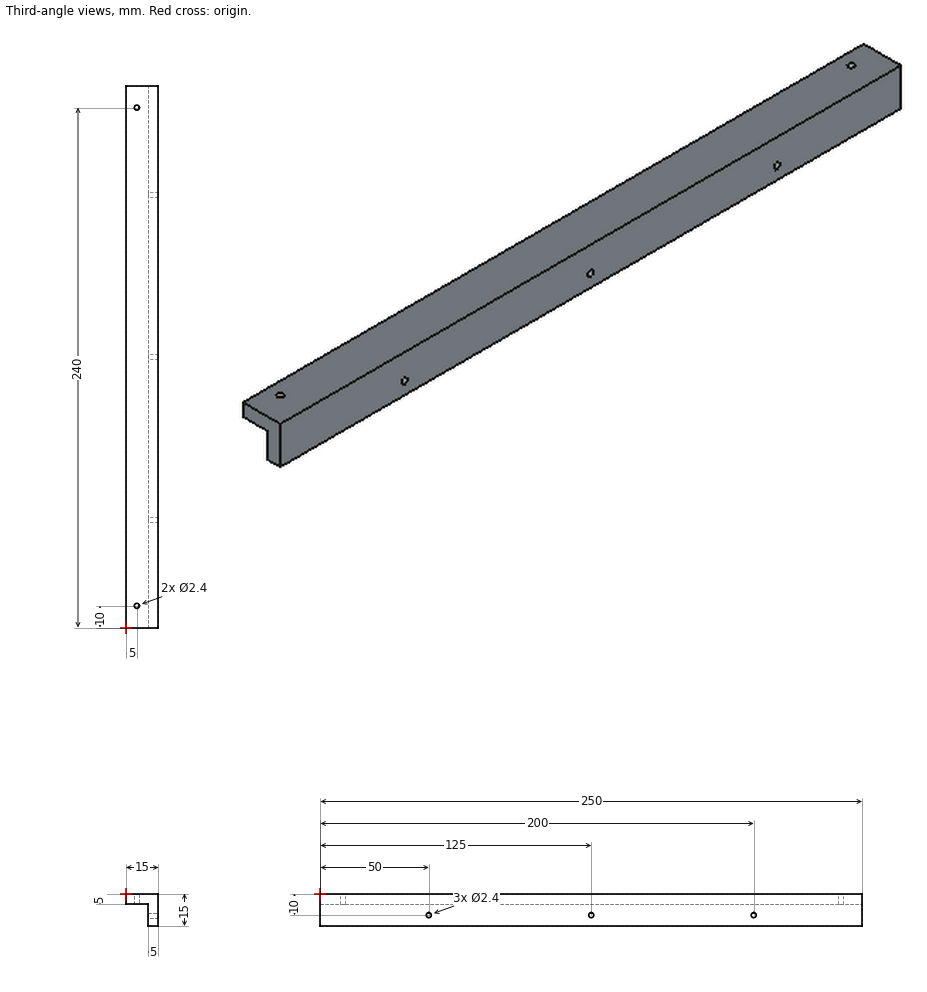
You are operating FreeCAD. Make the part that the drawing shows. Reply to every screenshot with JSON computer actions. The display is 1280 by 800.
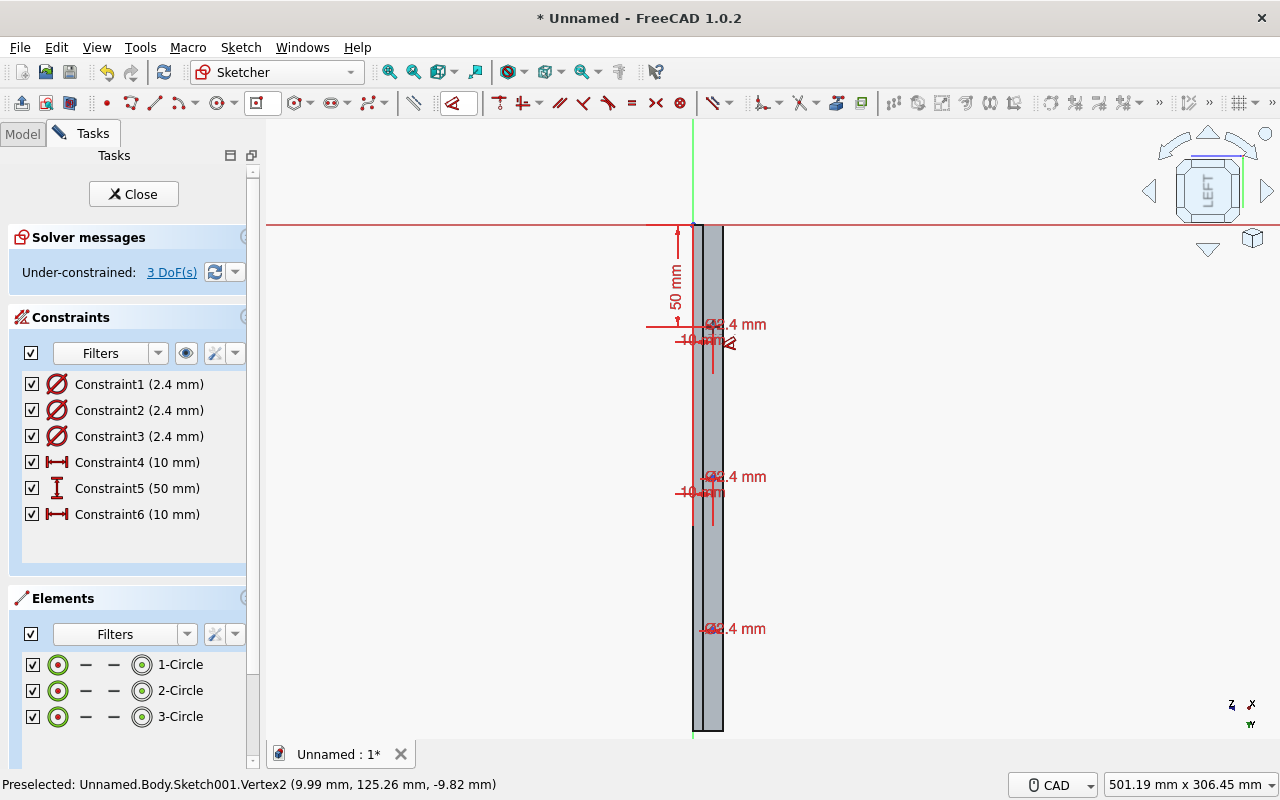
{"action": "scroll", "coordinate": [713, 631], "scroll_direction": "up", "scroll_amount": 4}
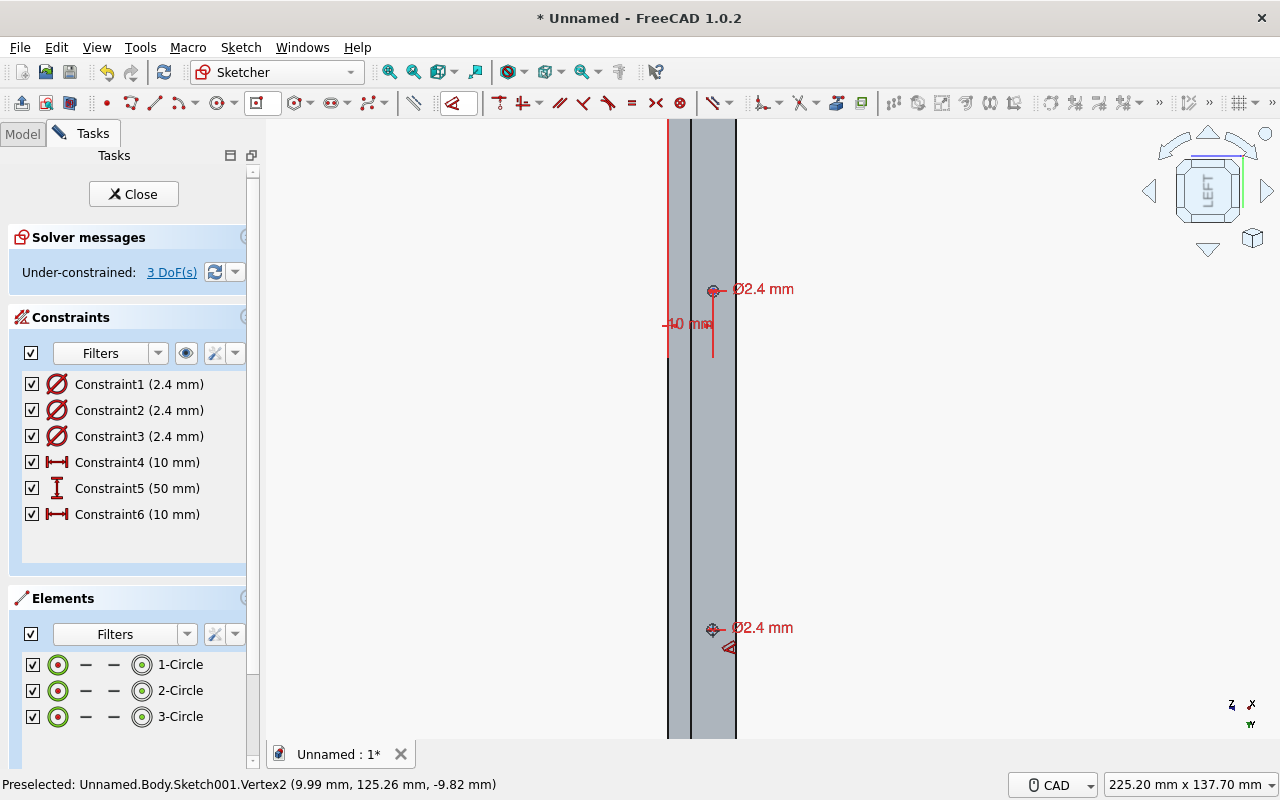
{"action": "left_click", "coordinate": [712, 630]}
{"action": "left_click", "coordinate": [690, 664]}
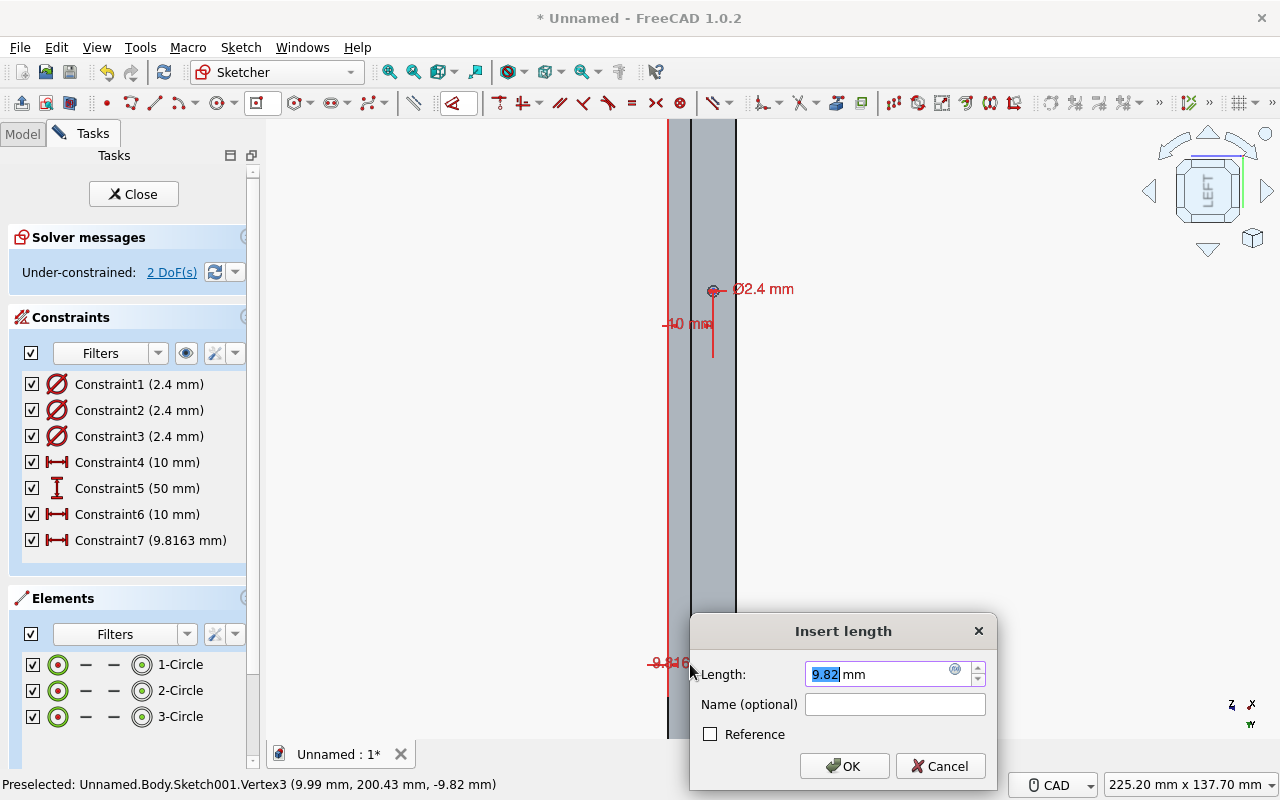
{"action": "type", "text": "10"}
{"action": "key", "text": "Return"}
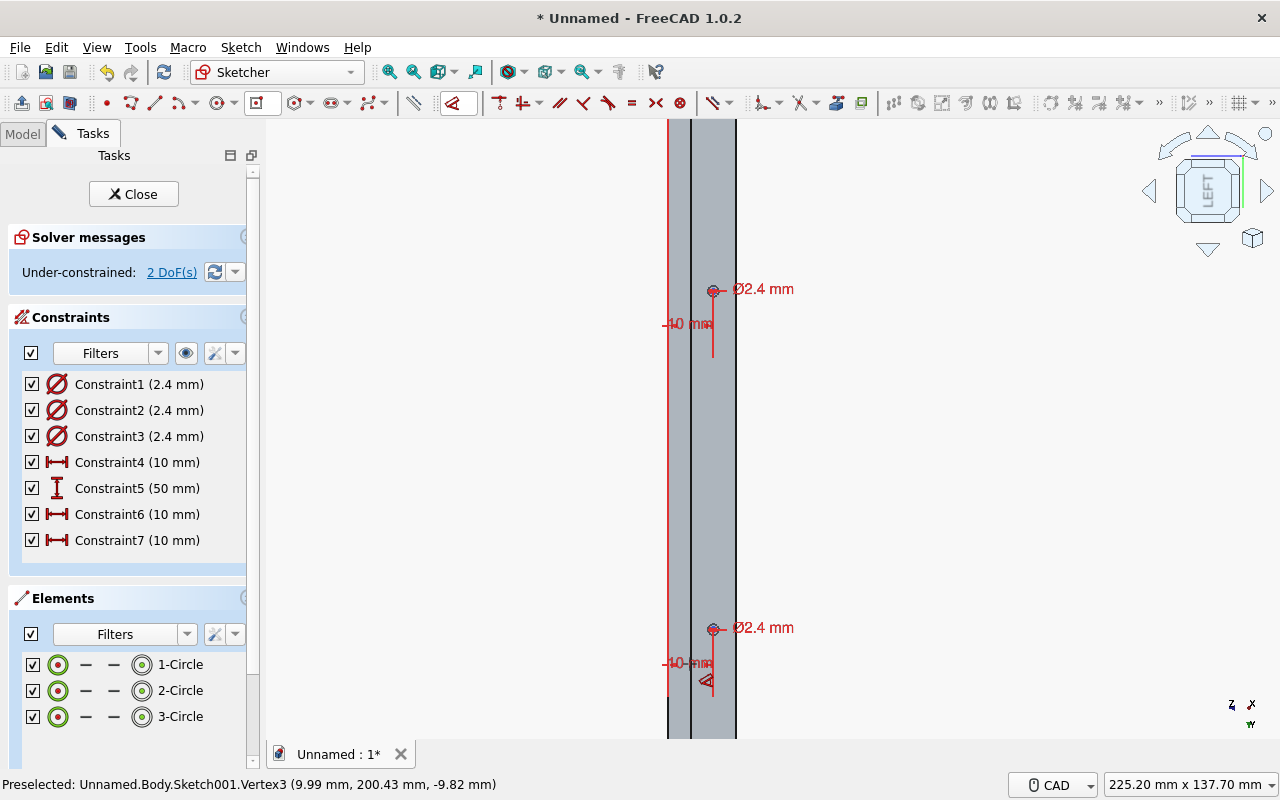
{"action": "left_click", "coordinate": [713, 291]}
{"action": "left_click", "coordinate": [634, 219]}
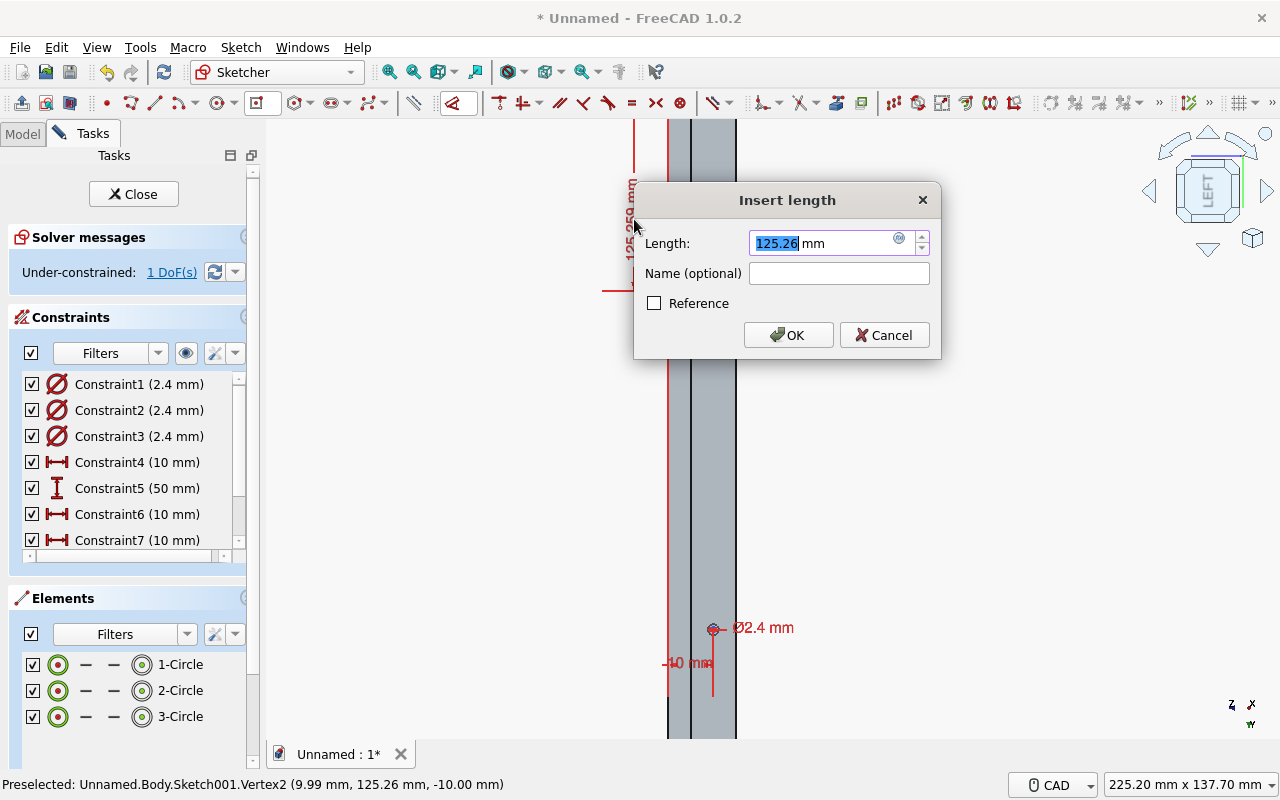
{"action": "type", "text": "125"}
{"action": "key", "text": "Return"}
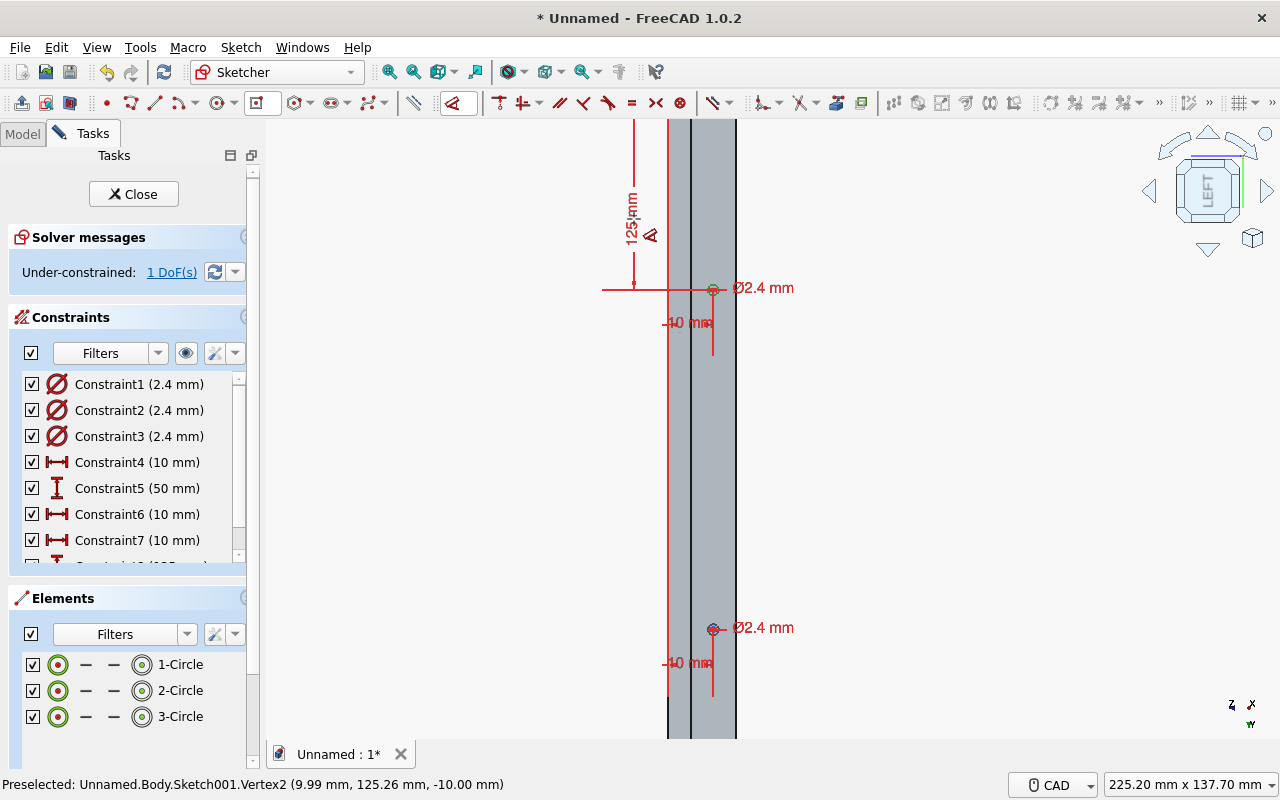
{"action": "left_click", "coordinate": [713, 630]}
{"action": "left_click", "coordinate": [634, 388]}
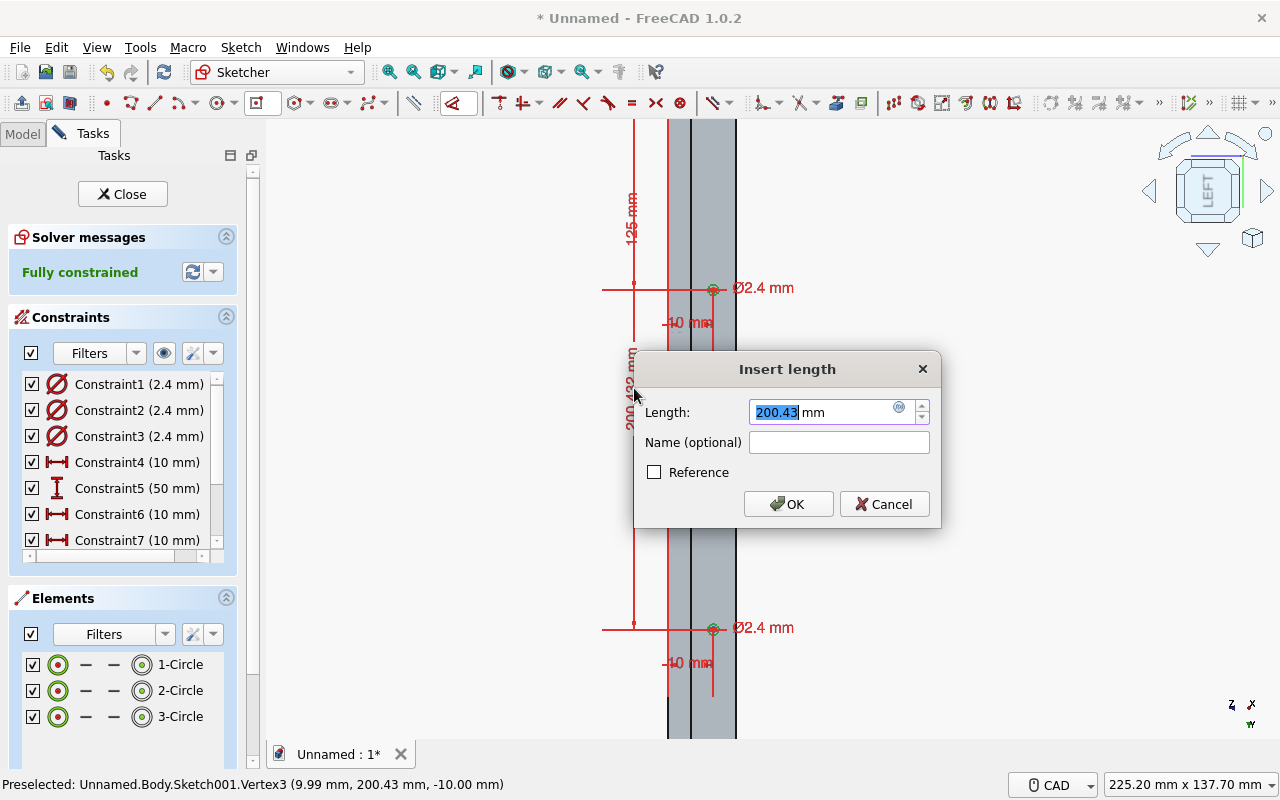
{"action": "type", "text": "200"}
{"action": "key", "text": "Return"}
{"action": "key", "text": "Escape"}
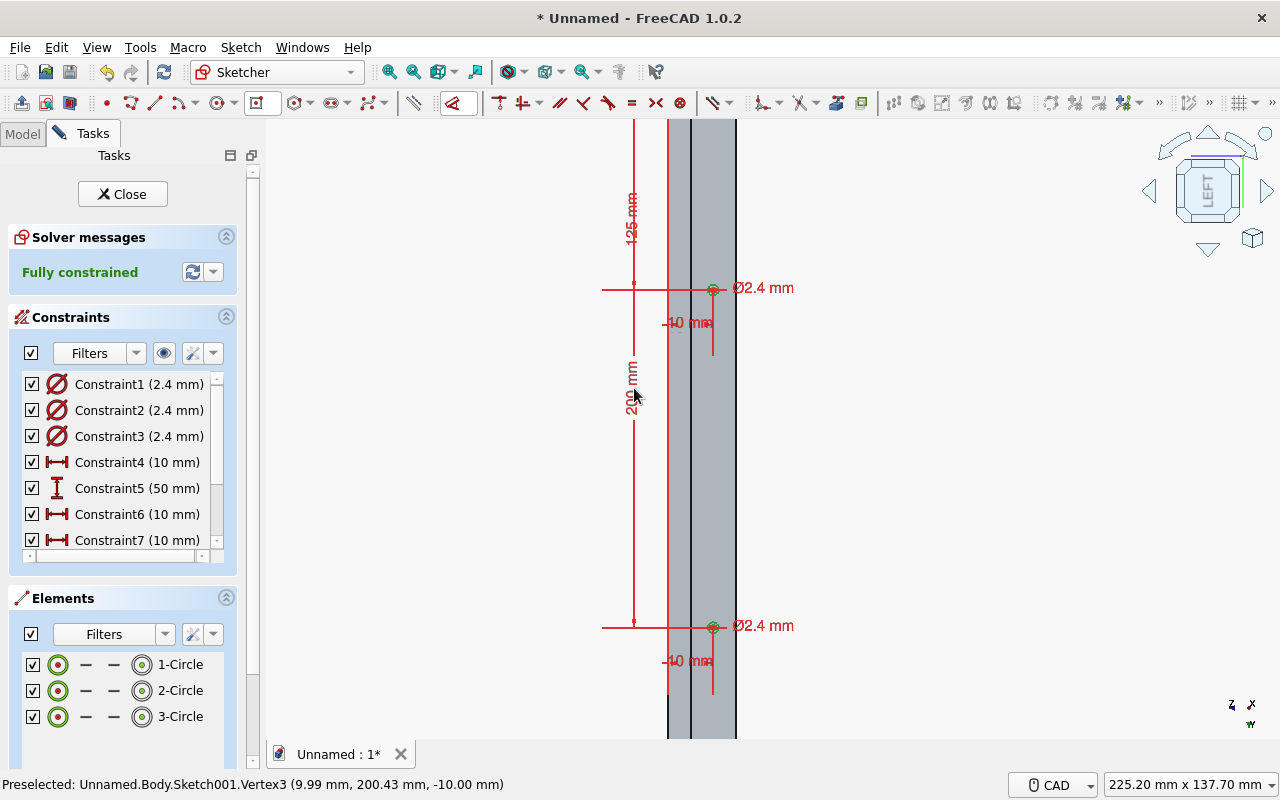
{"action": "left_click", "coordinate": [123, 194]}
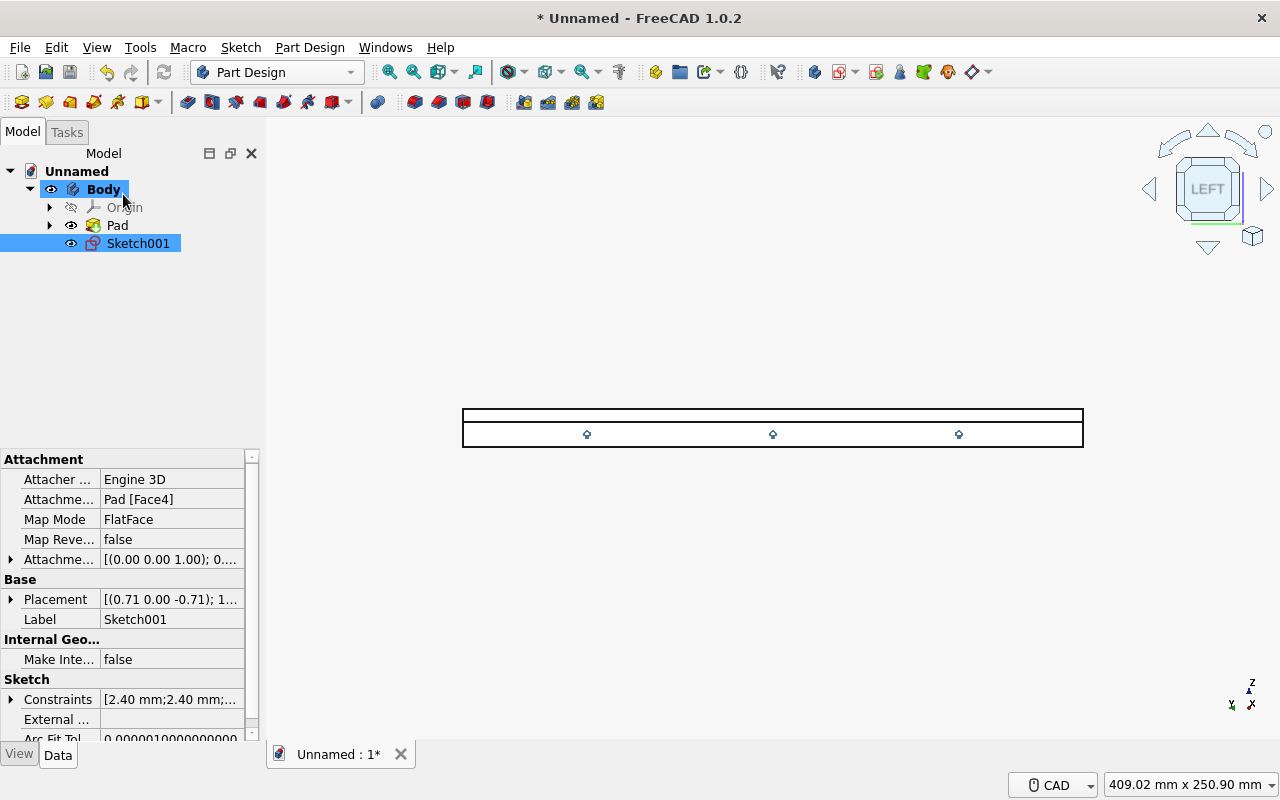
{"action": "left_click", "coordinate": [188, 102]}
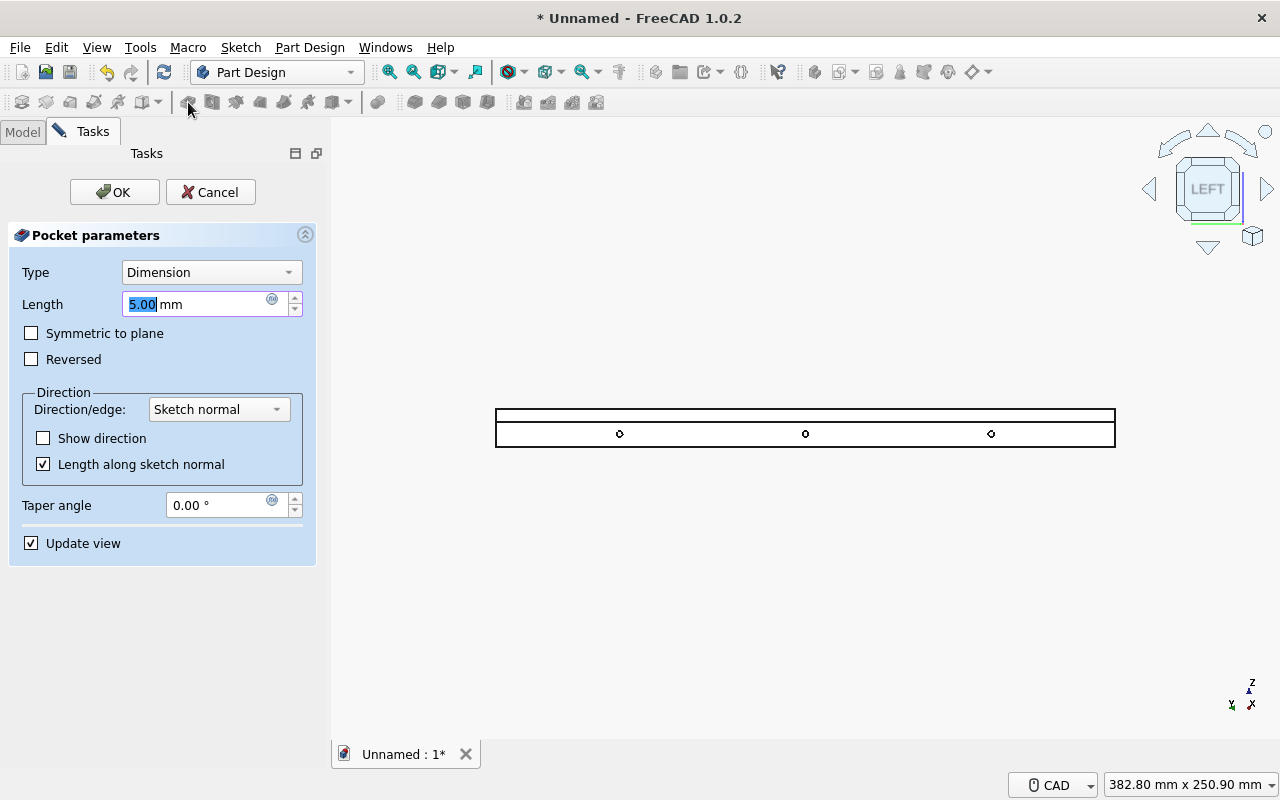
{"action": "type", "text": "10"}
{"action": "key", "text": "Tab"}